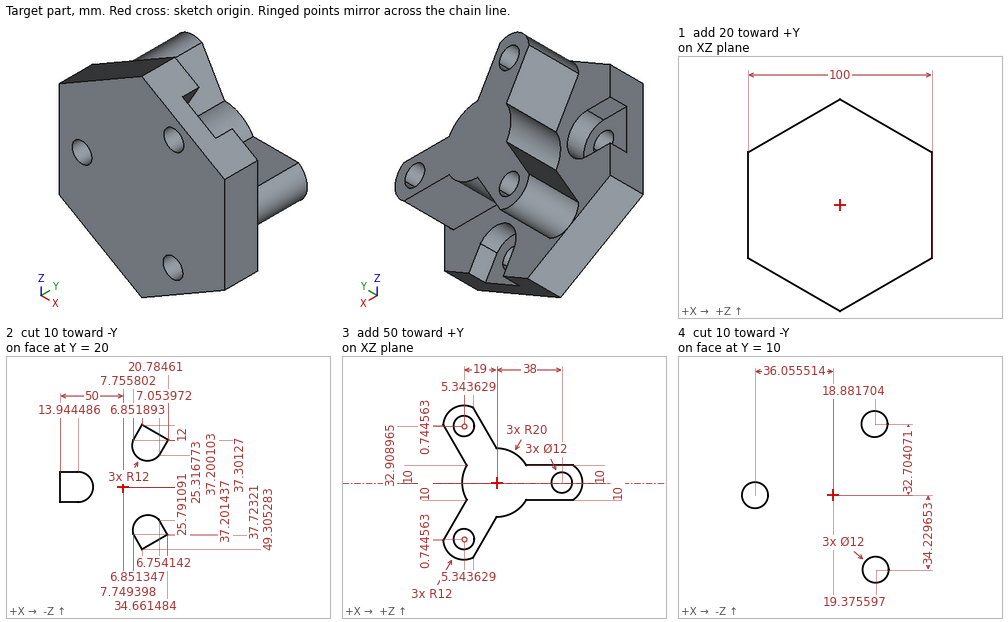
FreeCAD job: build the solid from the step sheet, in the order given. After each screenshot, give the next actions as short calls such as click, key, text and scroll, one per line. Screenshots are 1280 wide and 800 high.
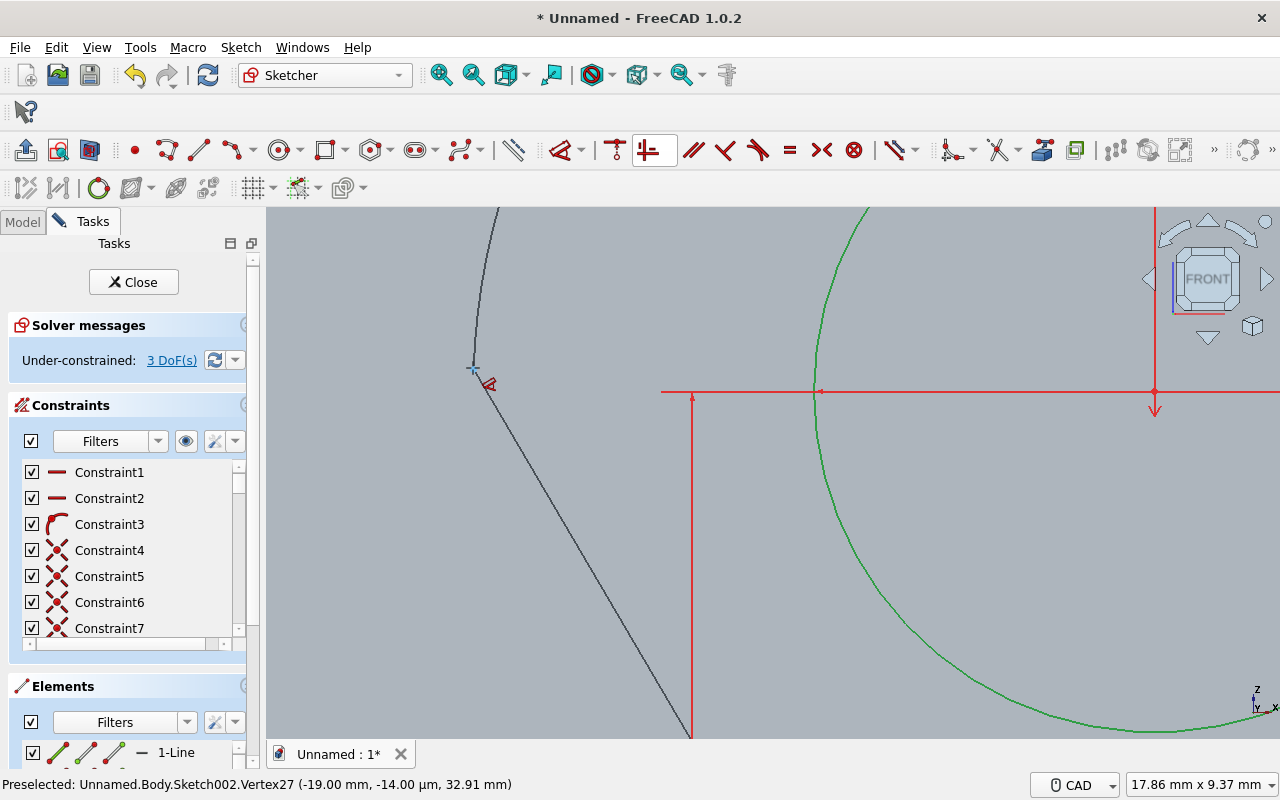
click(474, 369)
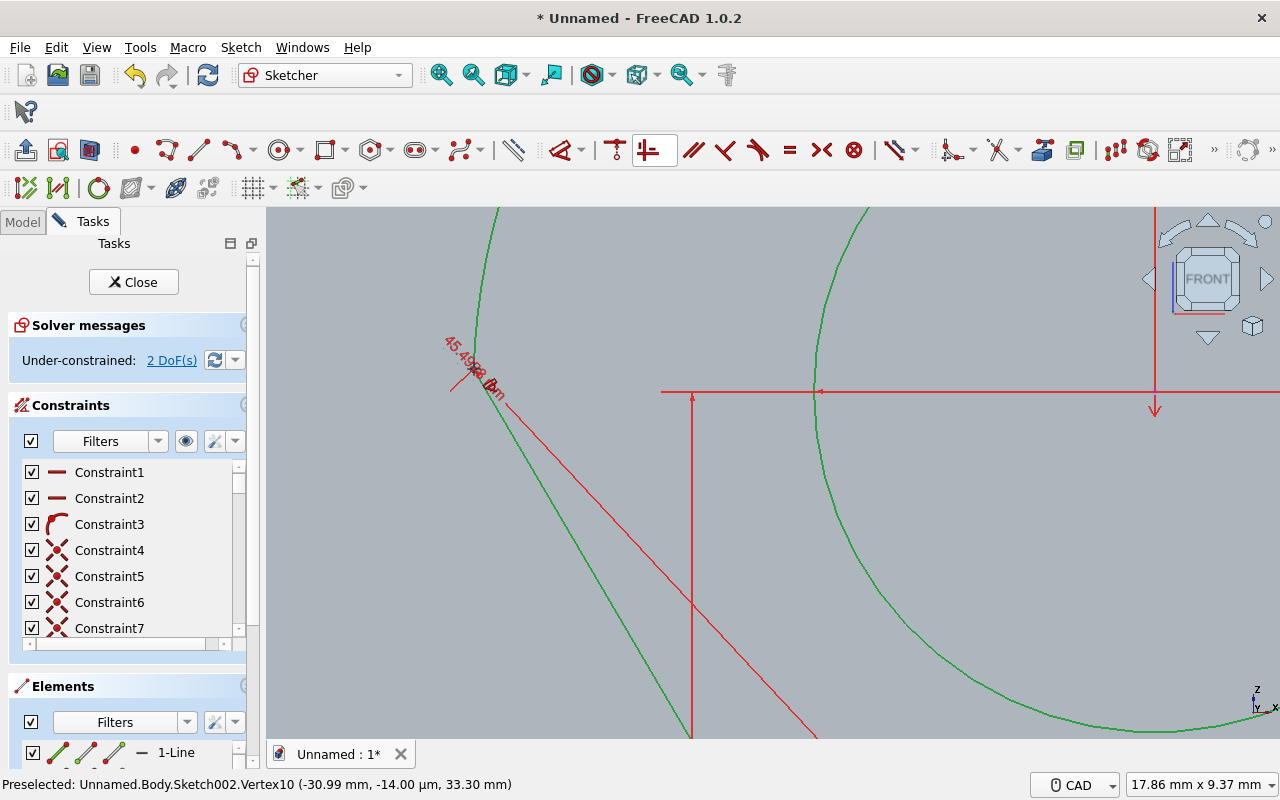
scroll(538, 330, down, 13)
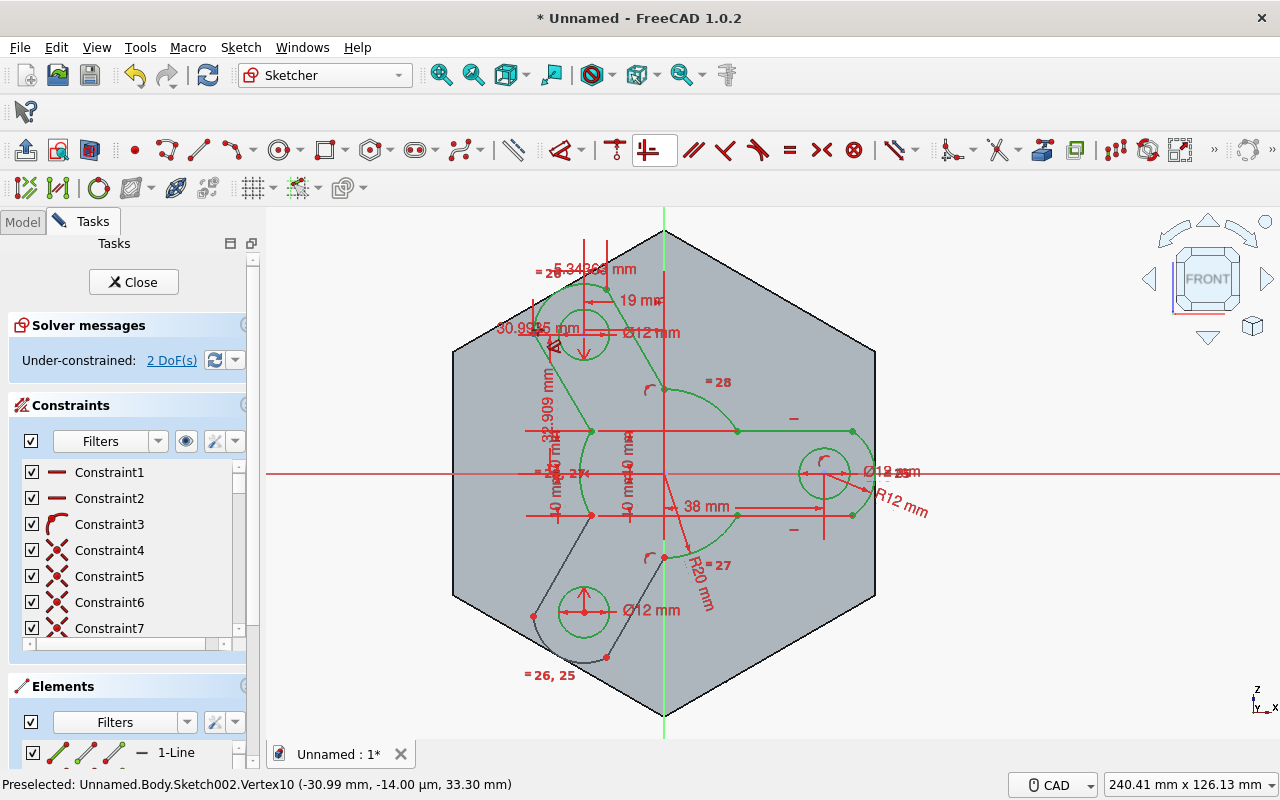
scroll(584, 335, up, 13)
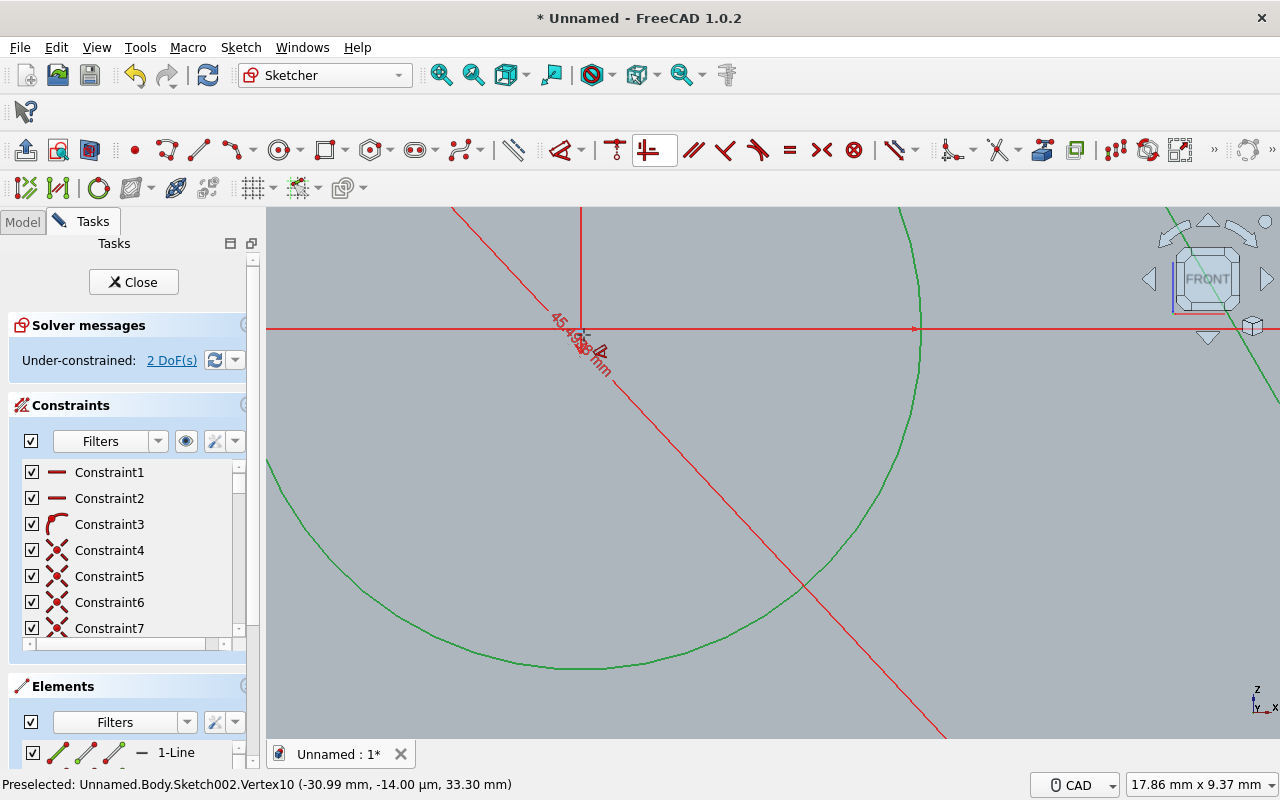
click(581, 329)
click(615, 318)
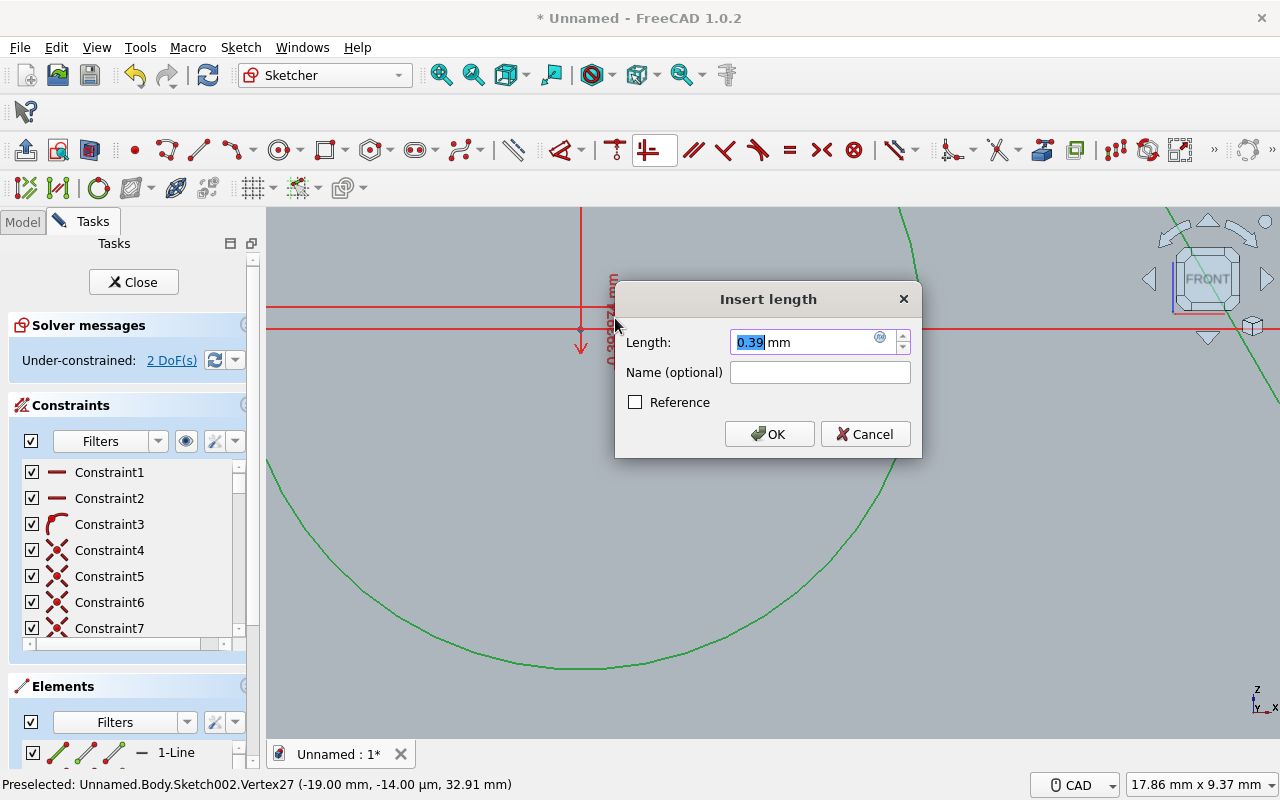
text(0.744563)
key(Return)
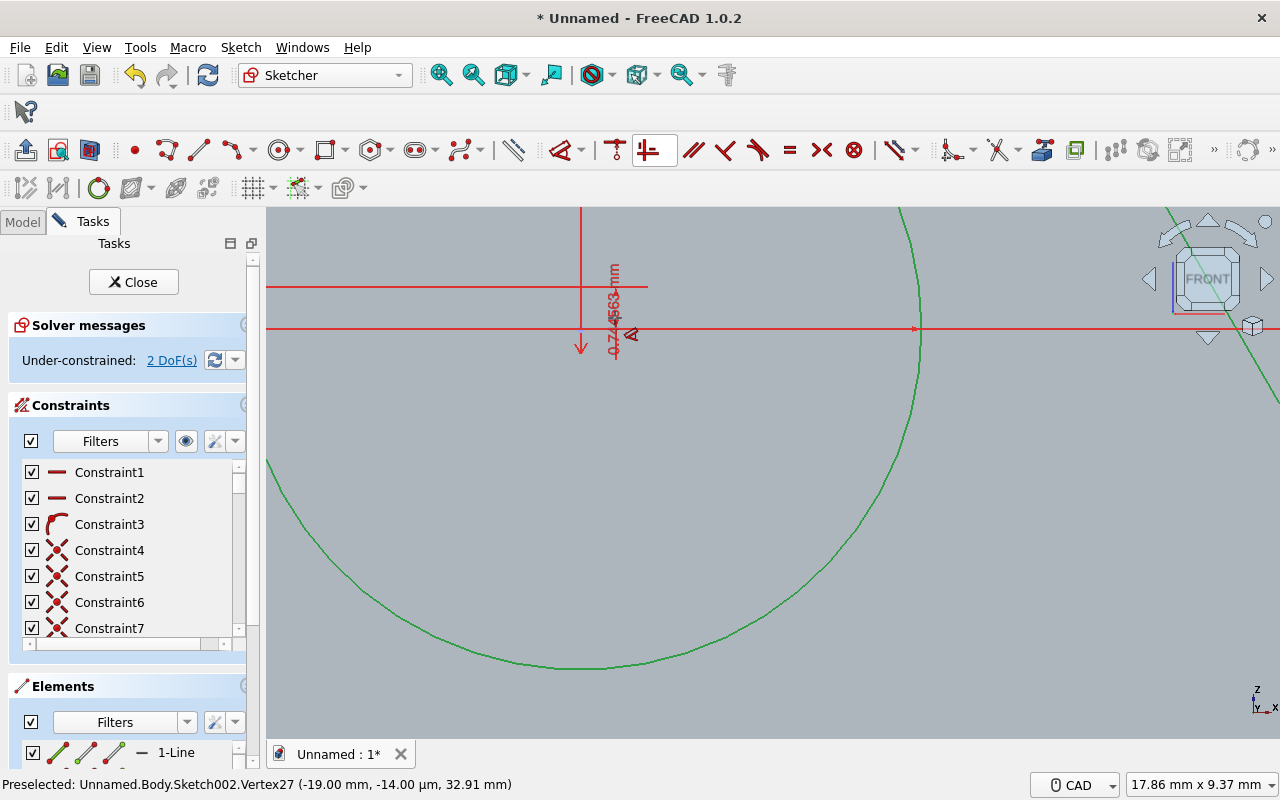
scroll(585, 335, down, 13)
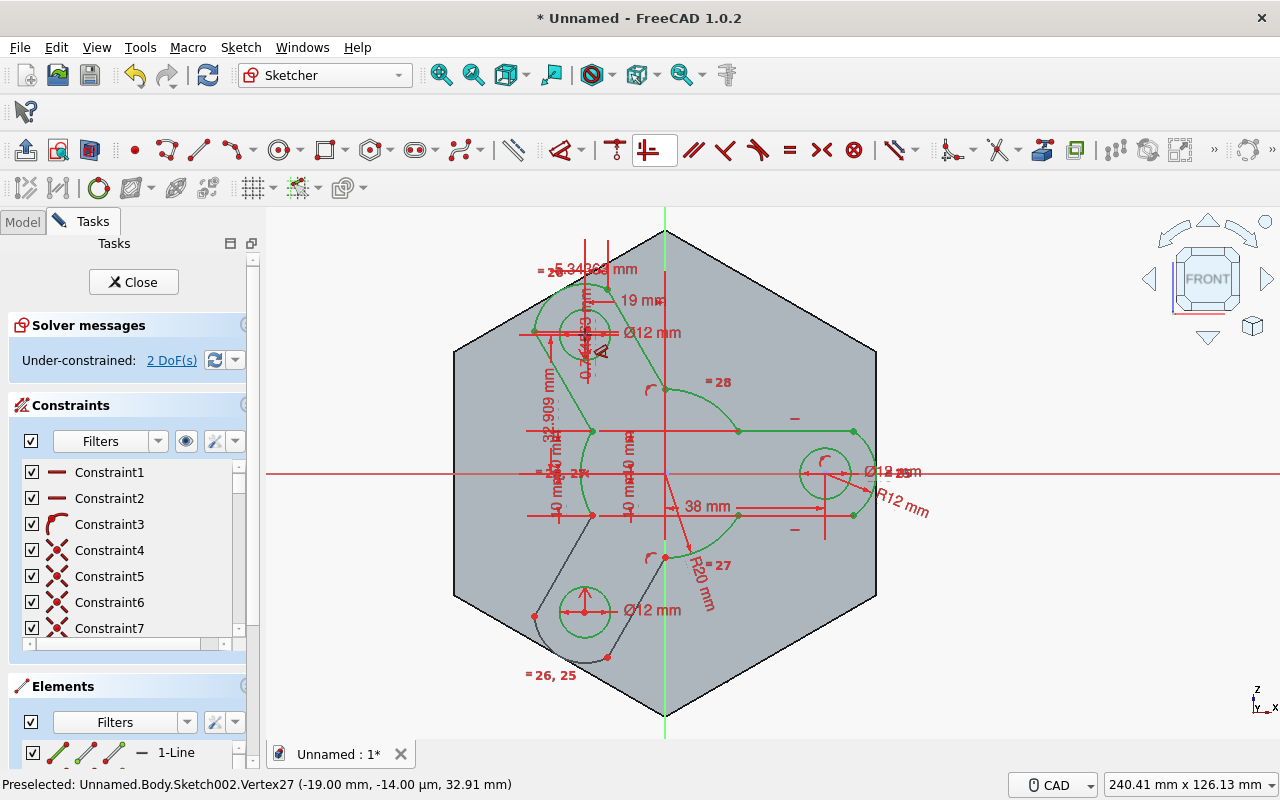
scroll(608, 658, up, 3)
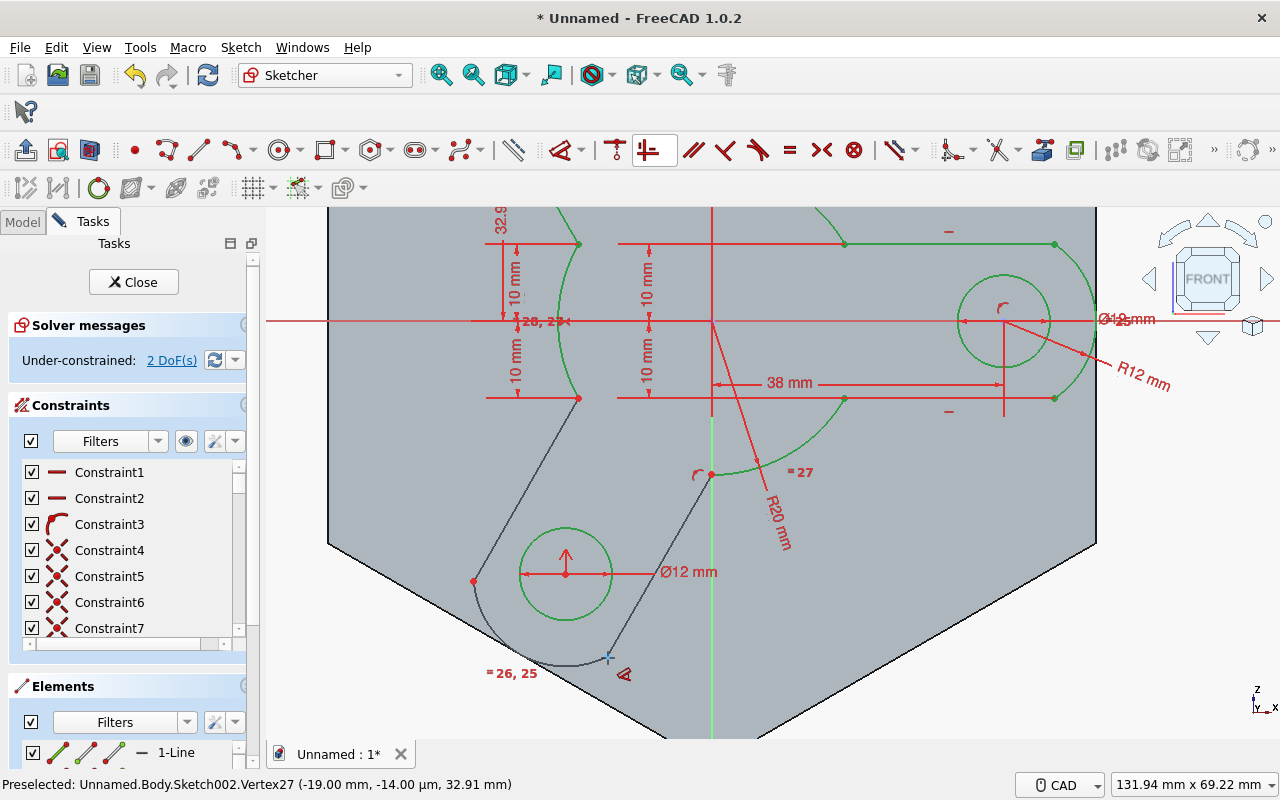
click(607, 657)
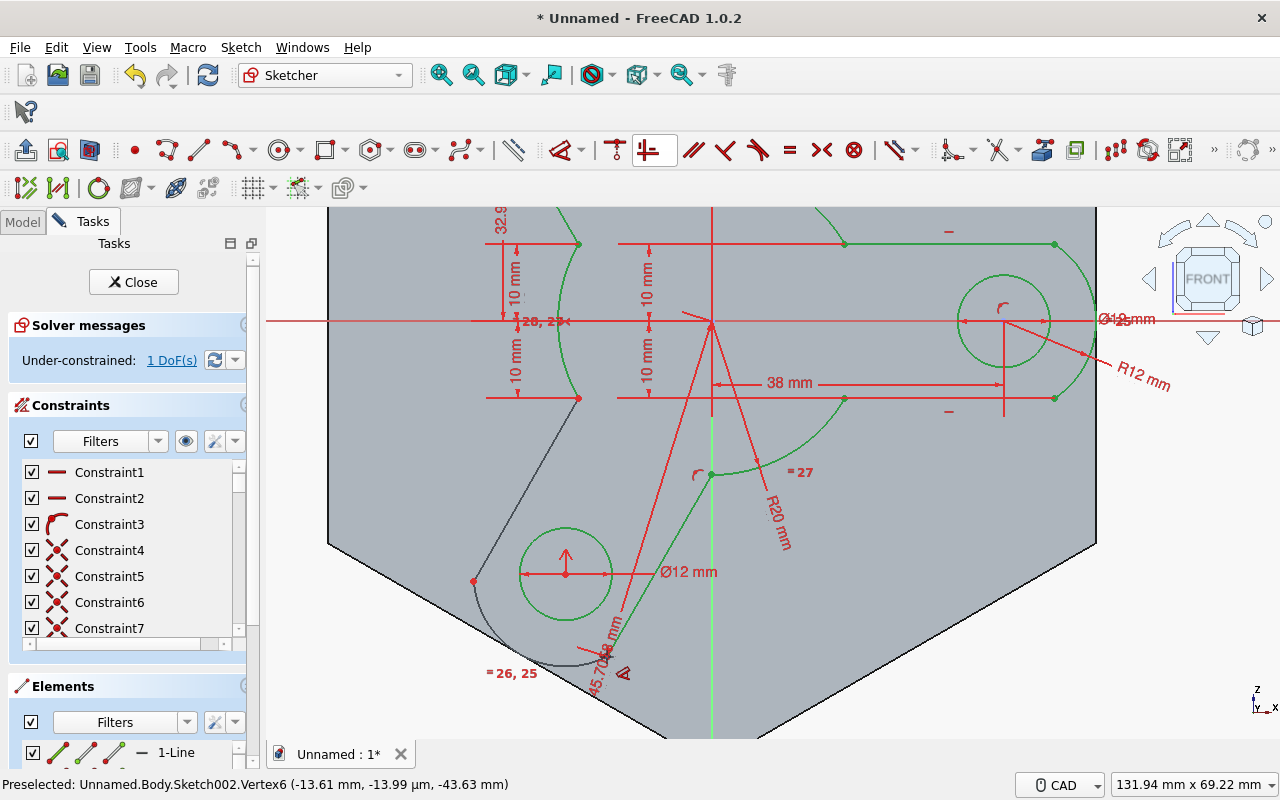
click(566, 574)
click(586, 691)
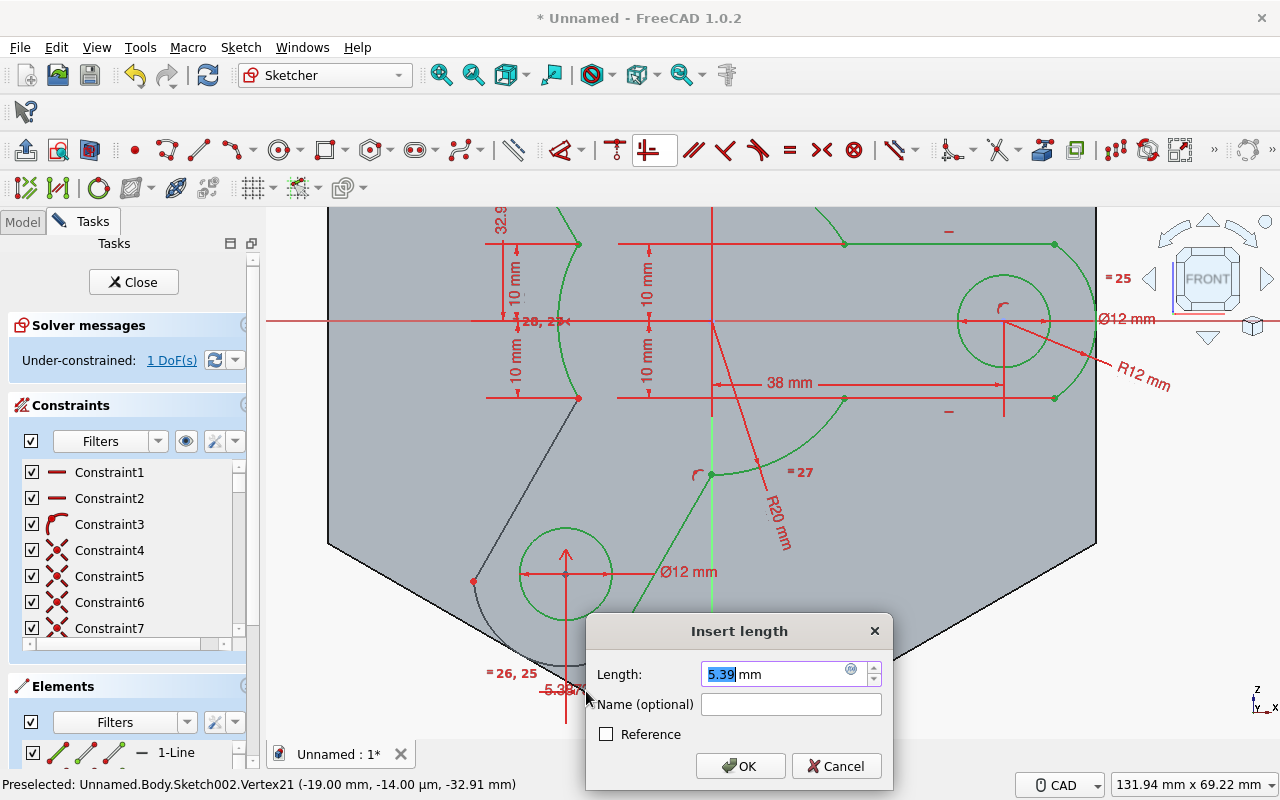
text(5.343629)
key(Return)